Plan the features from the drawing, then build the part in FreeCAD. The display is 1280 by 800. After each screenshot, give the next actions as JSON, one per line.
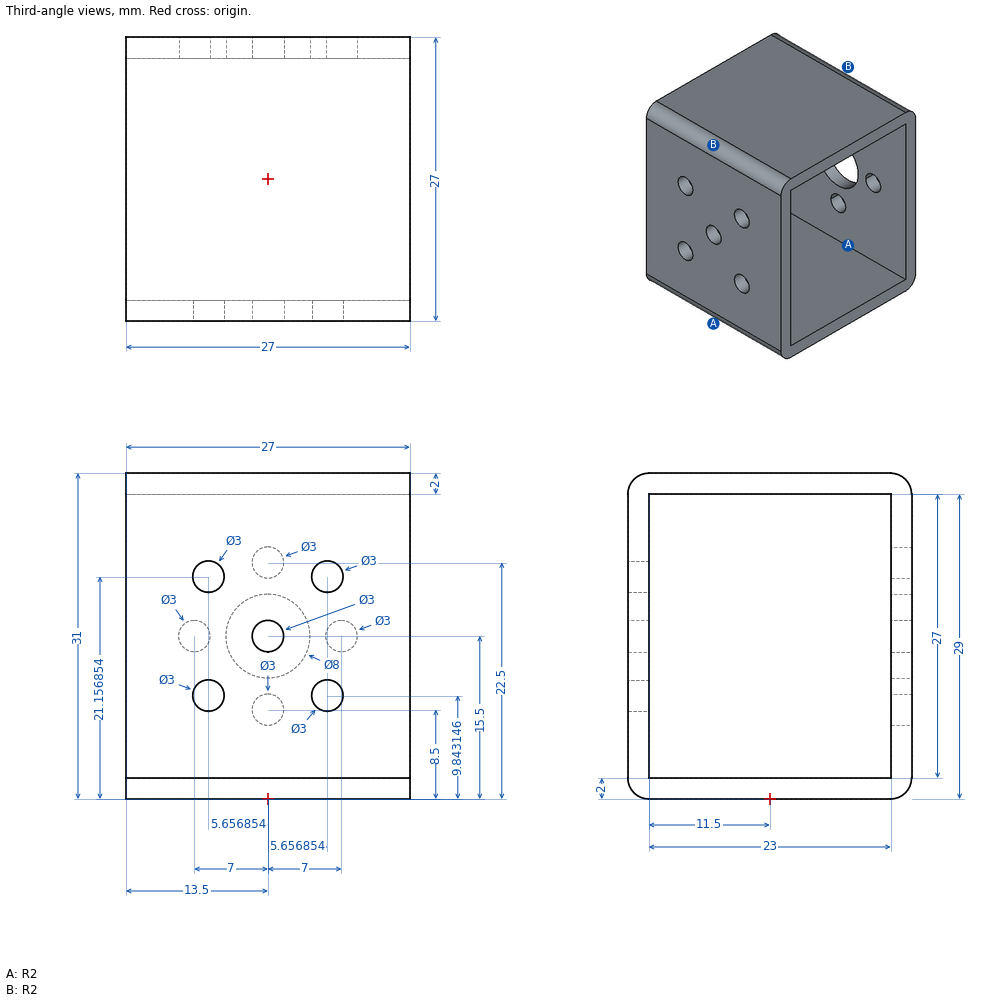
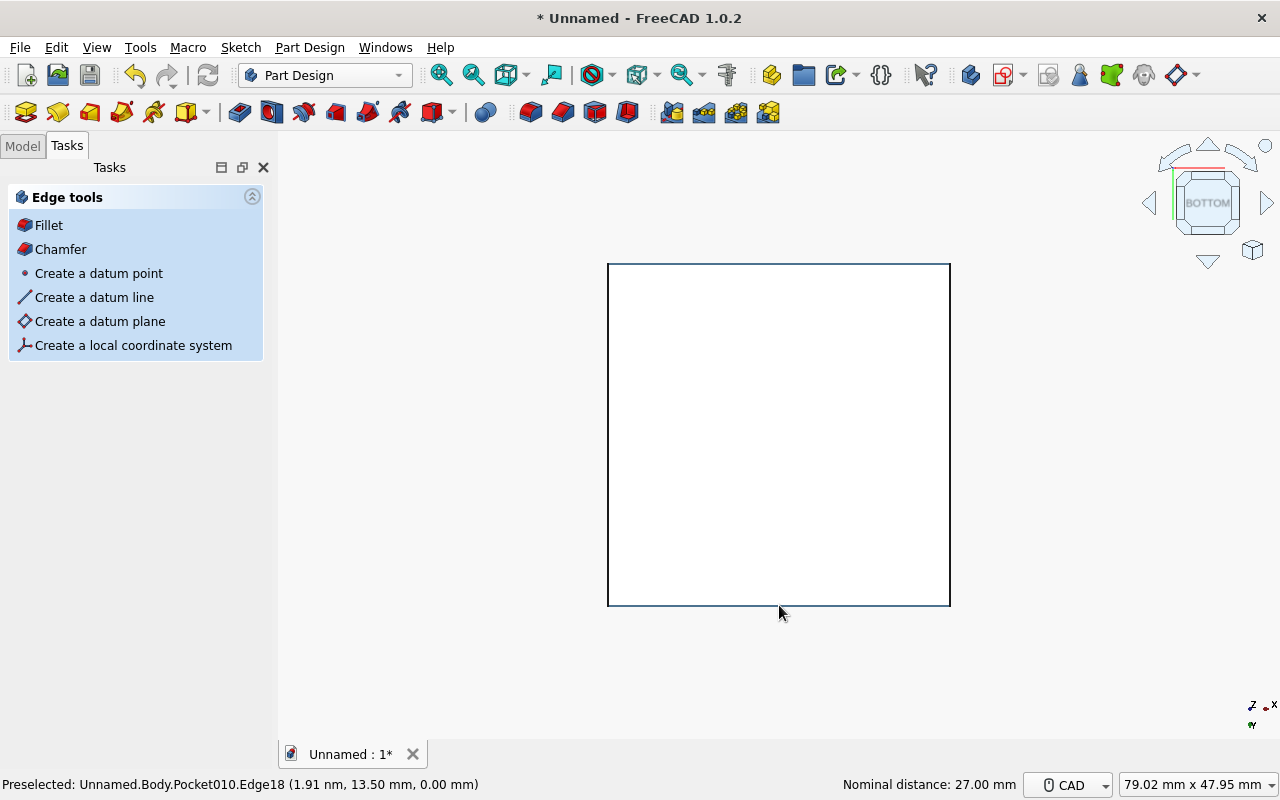
{"action": "left_click", "coordinate": [532, 112]}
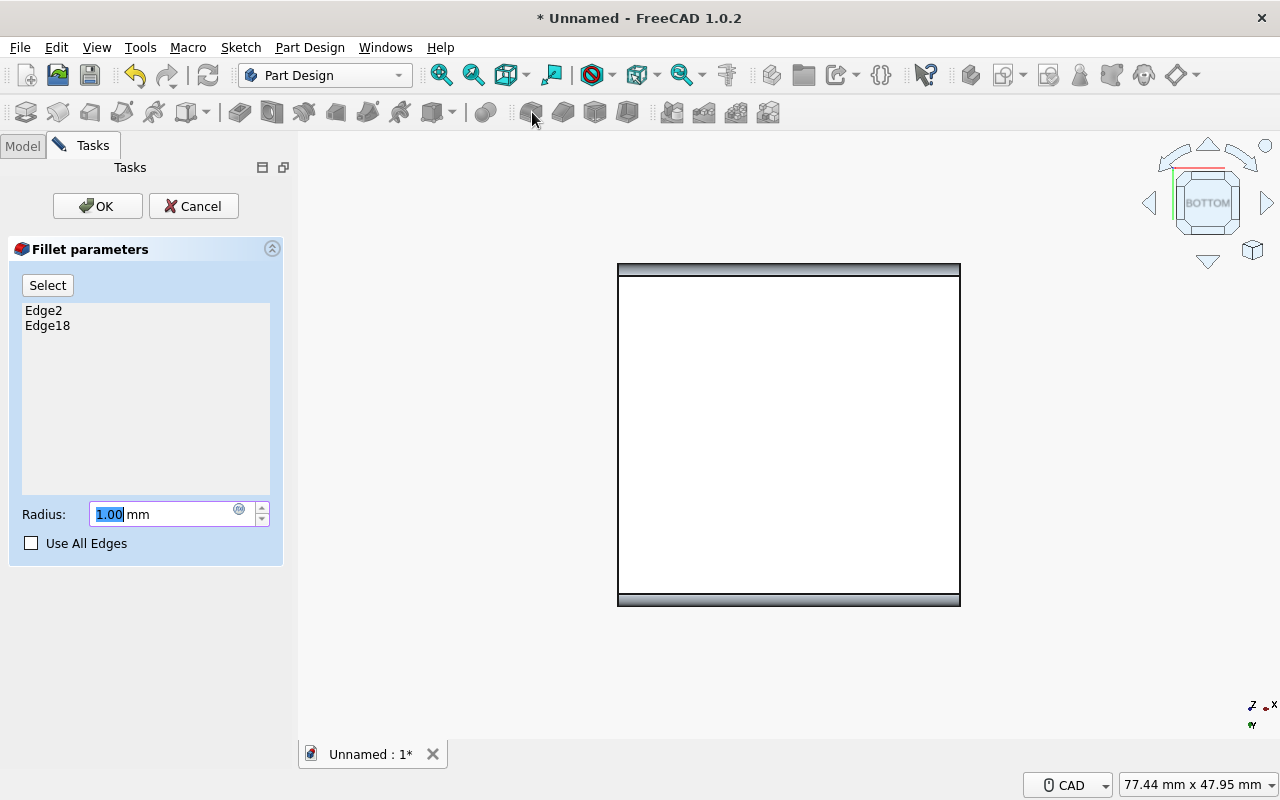
{"action": "type", "text": "2"}
{"action": "key", "text": "Tab"}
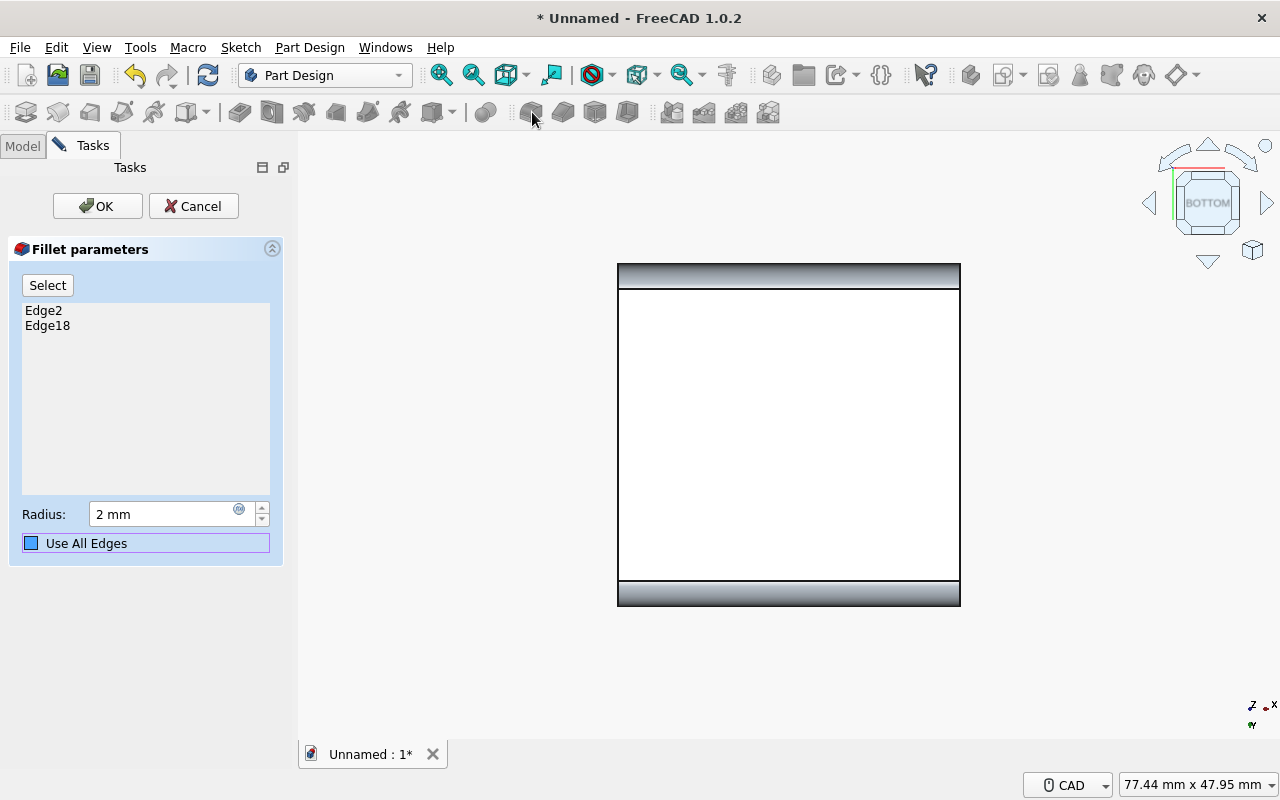
{"action": "left_click", "coordinate": [98, 206]}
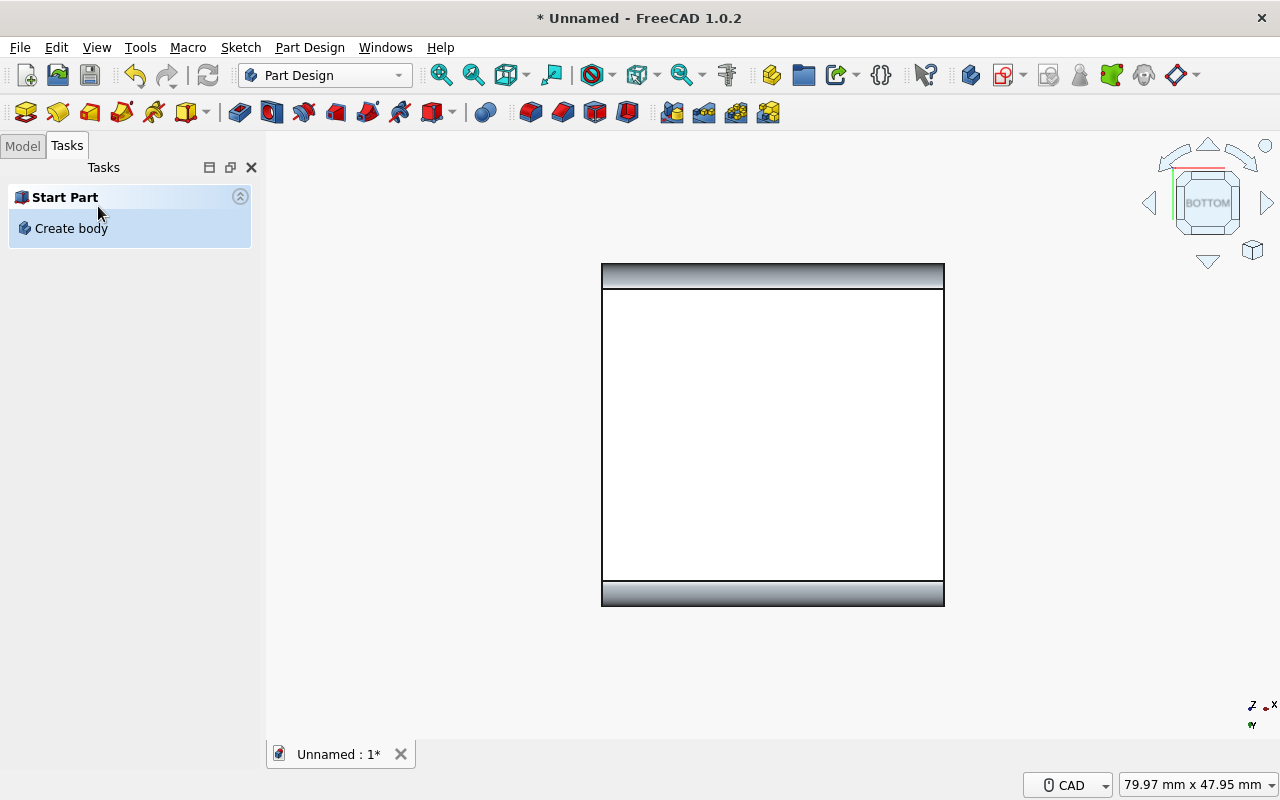
{"action": "key", "text": "0"}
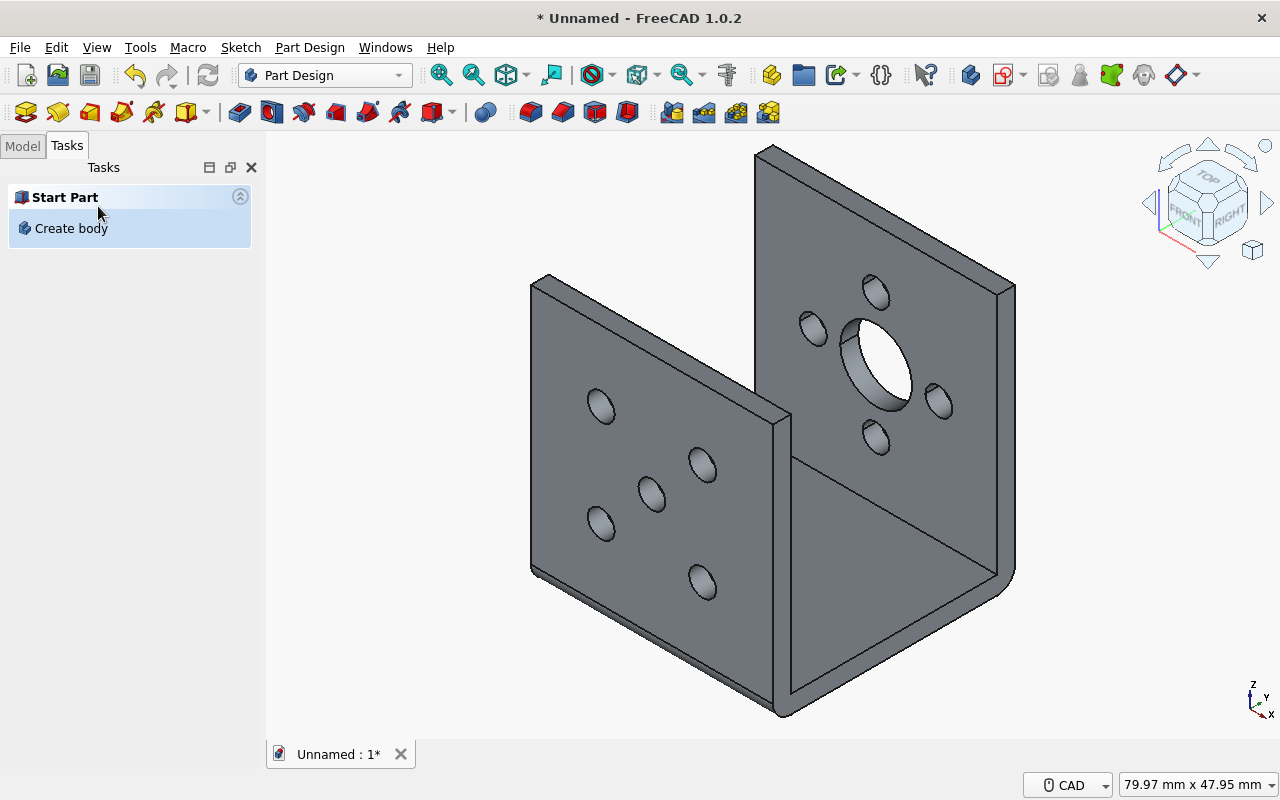
{"action": "left_click", "coordinate": [652, 414]}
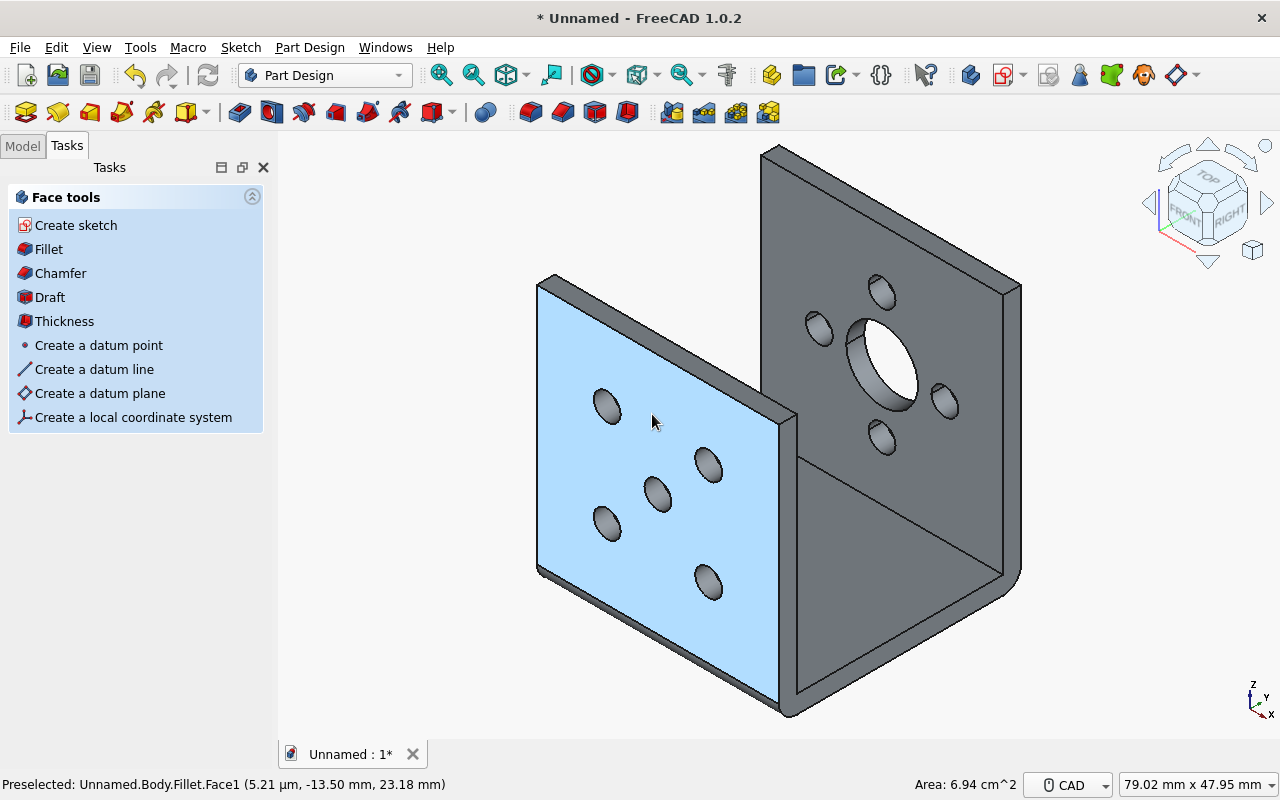
{"action": "left_click", "coordinate": [1004, 76]}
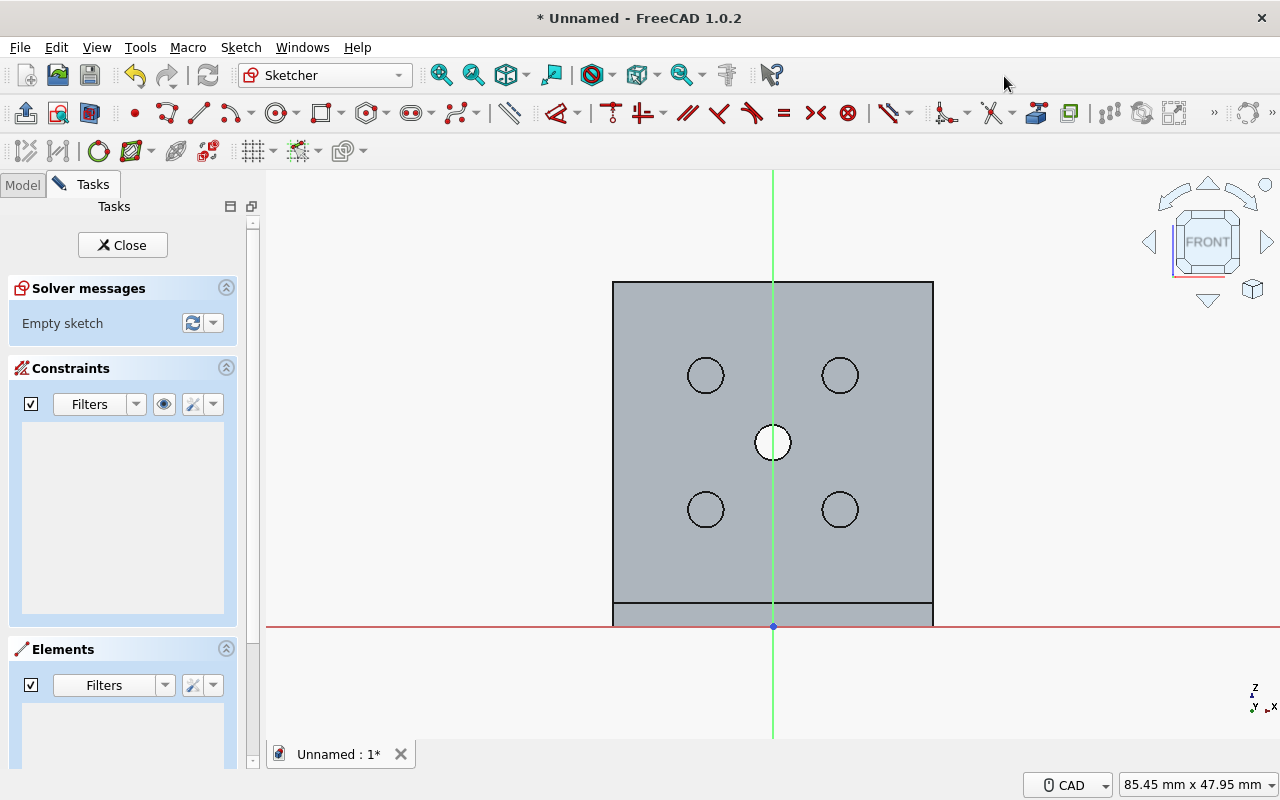
{"action": "key", "text": "g r"}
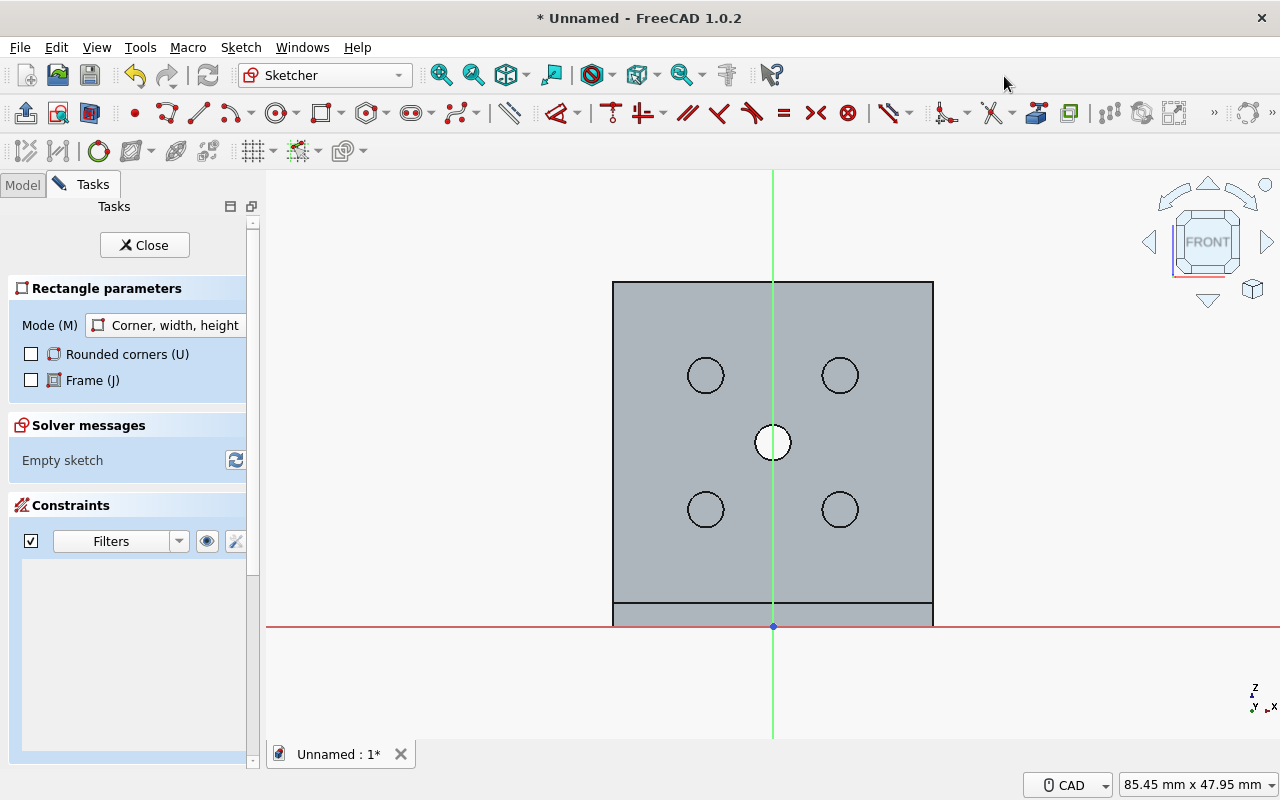
{"action": "left_click", "coordinate": [613, 259]}
{"action": "mouse_move", "coordinate": [933, 282]}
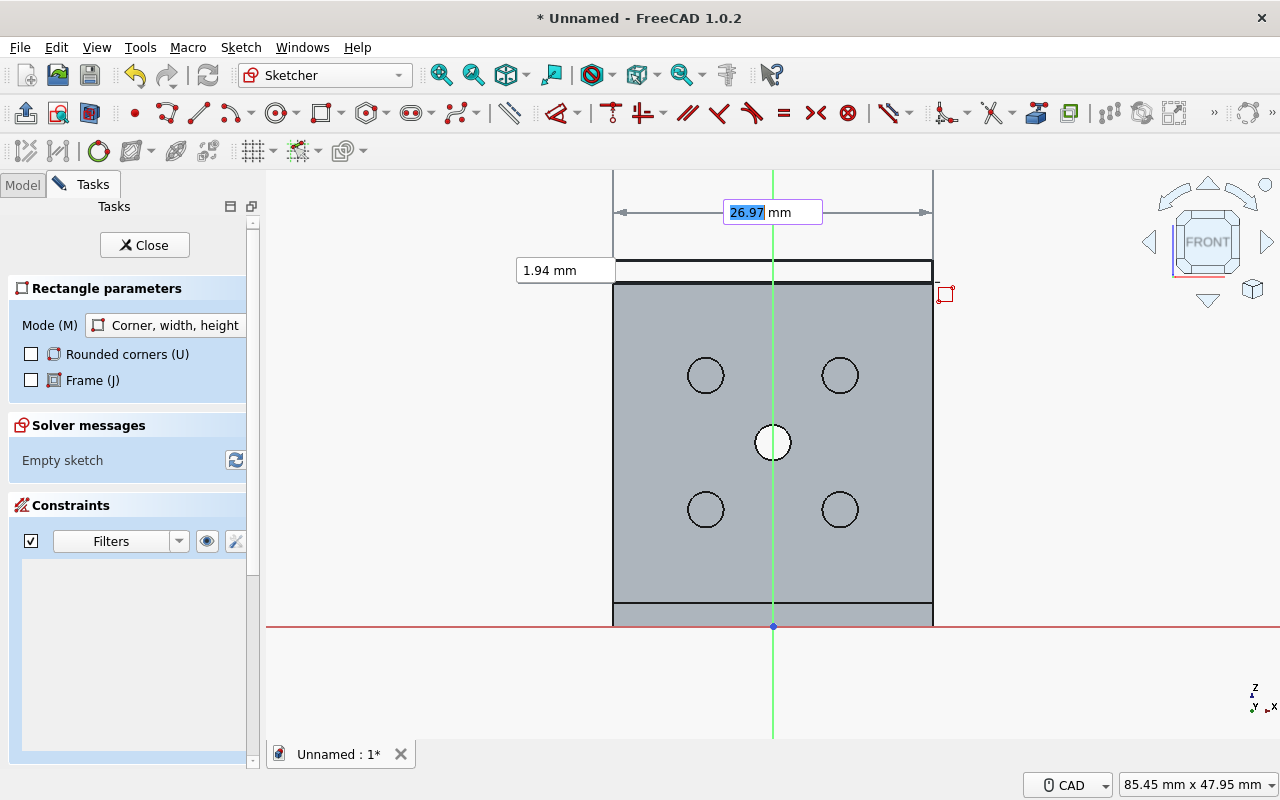
{"action": "type", "text": "27"}
{"action": "key", "text": "Tab"}
{"action": "type", "text": "2"}
{"action": "key", "text": "Return"}
{"action": "key", "text": "Escape"}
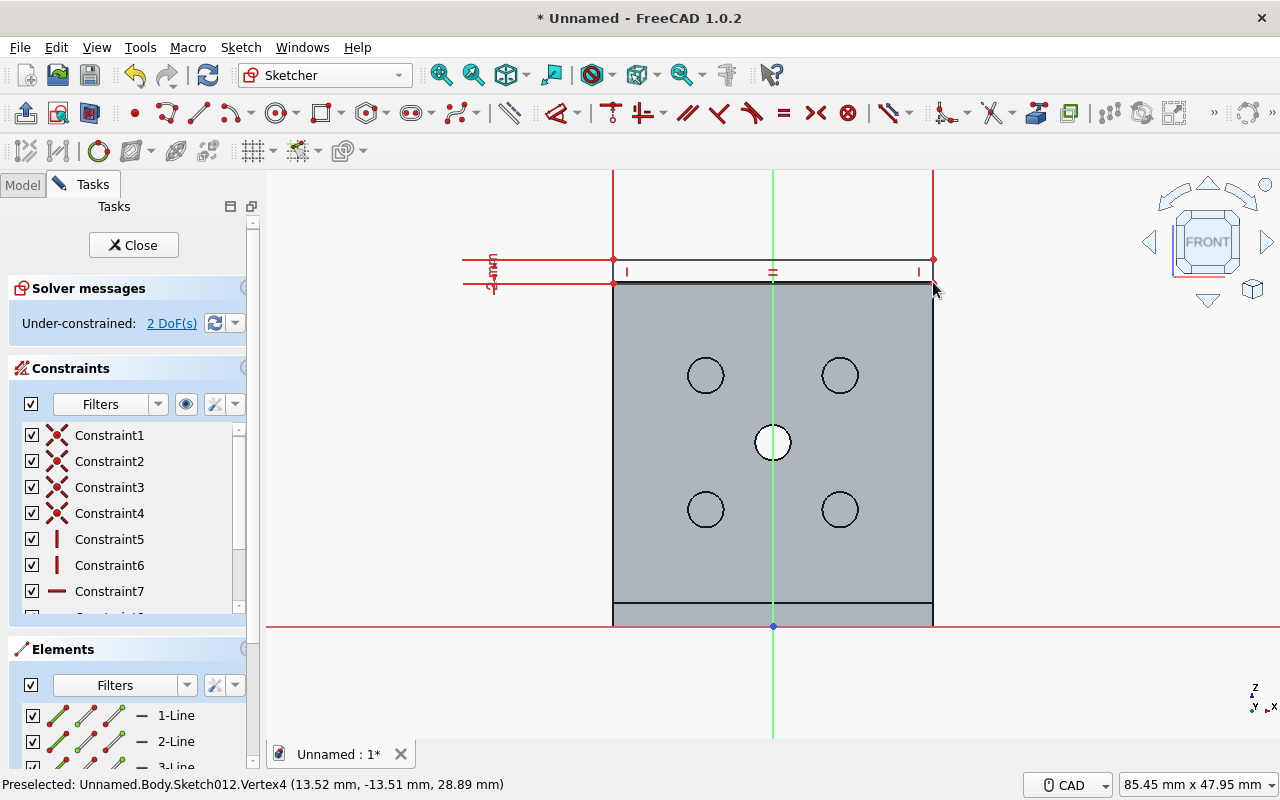
{"action": "left_click", "coordinate": [556, 114]}